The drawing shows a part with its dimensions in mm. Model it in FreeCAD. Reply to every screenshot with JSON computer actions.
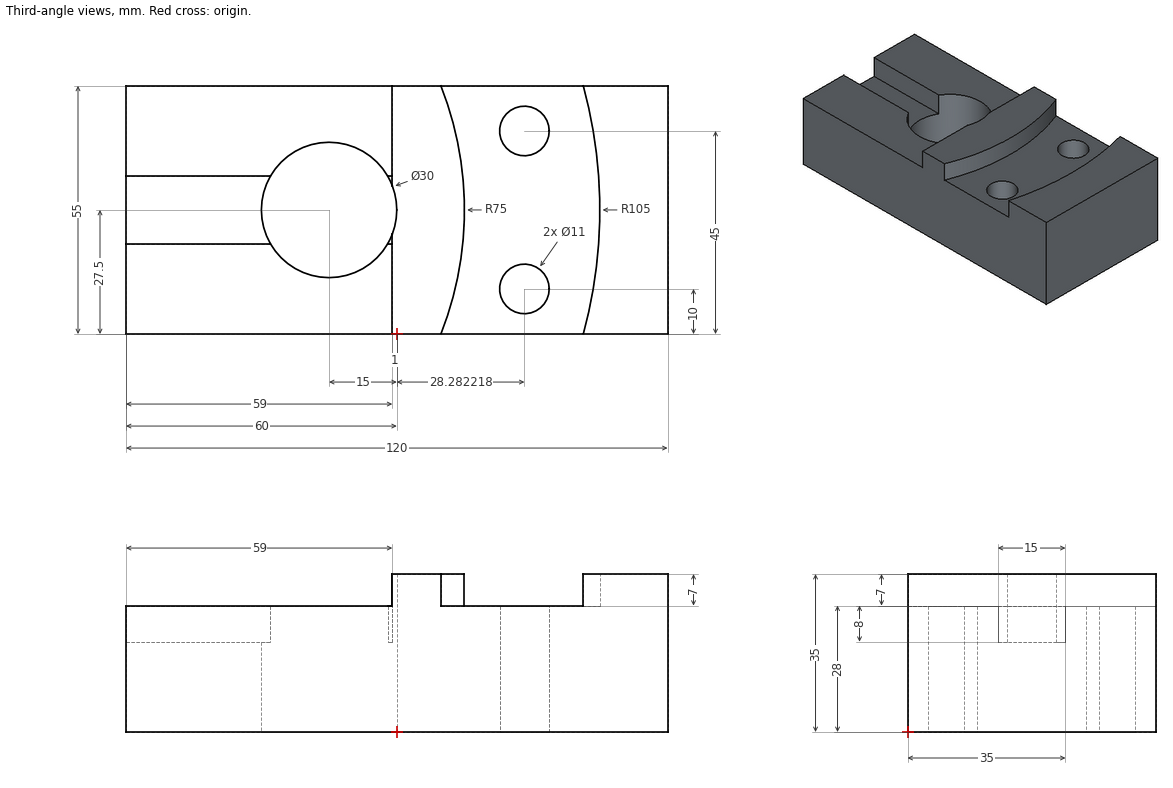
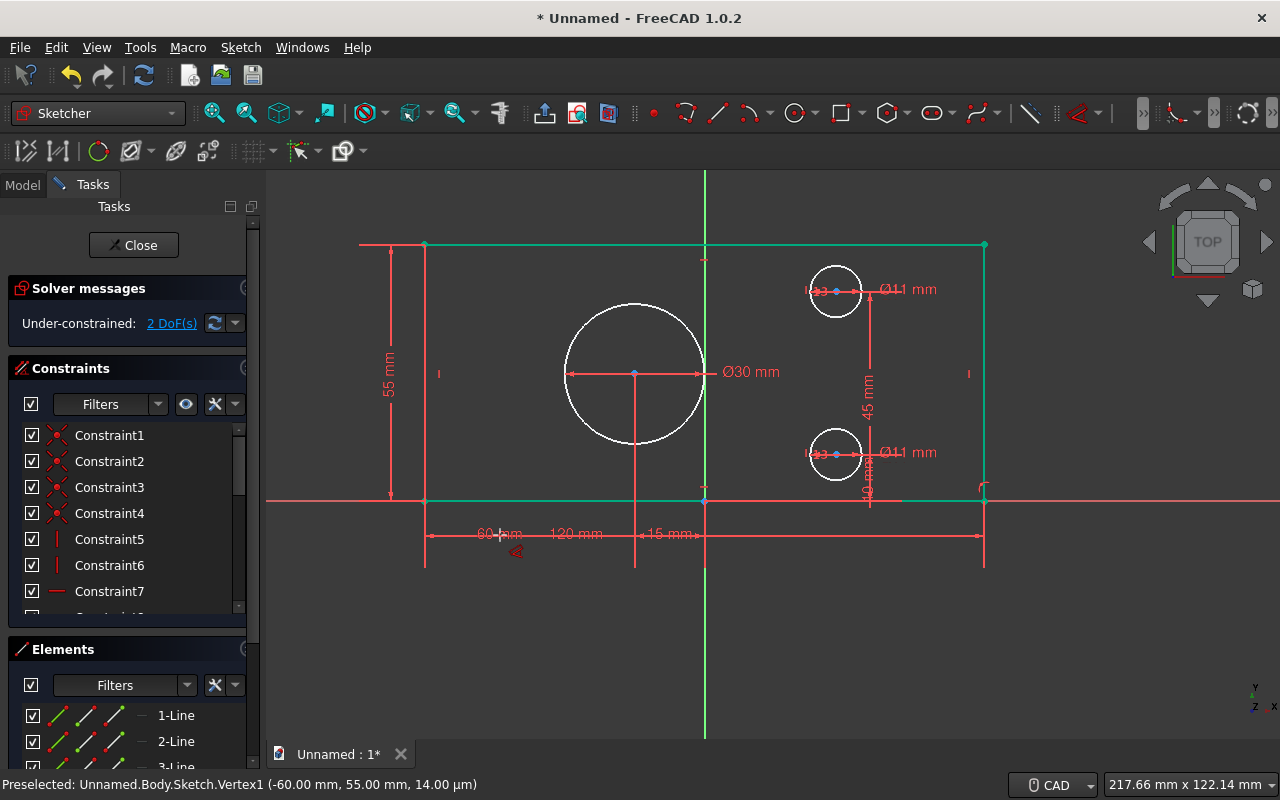
{"action": "left_click", "coordinate": [635, 374]}
{"action": "left_click", "coordinate": [601, 408]}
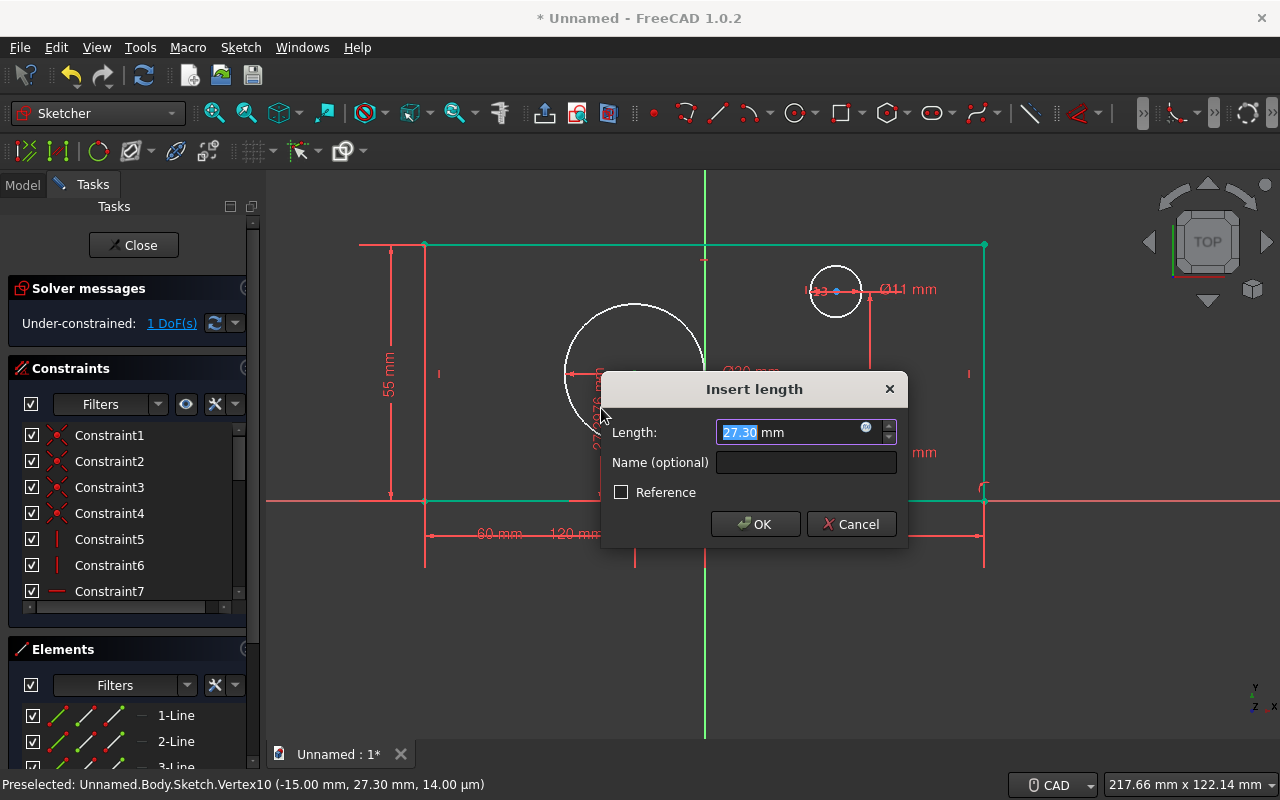
{"action": "type", "text": "27.5"}
{"action": "key", "text": "Return"}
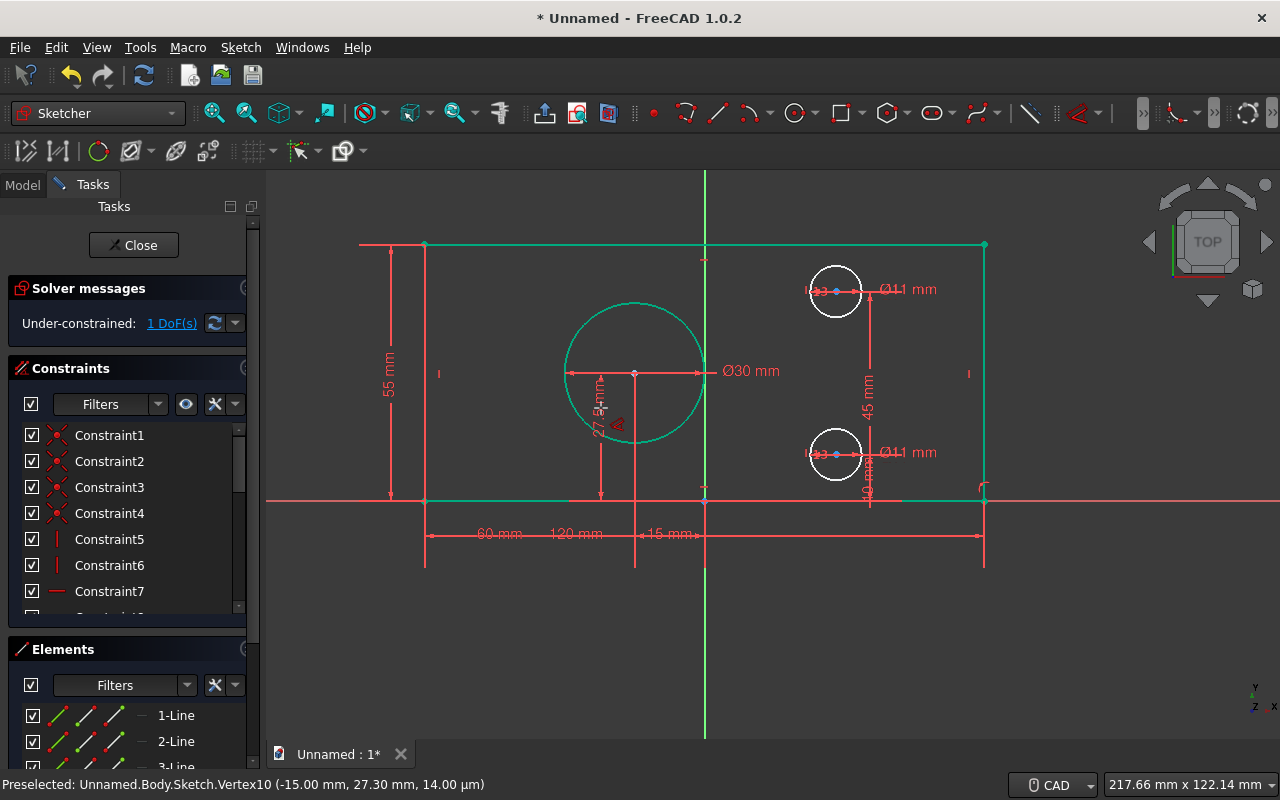
{"action": "left_click", "coordinate": [836, 455]}
{"action": "left_click", "coordinate": [770, 535]}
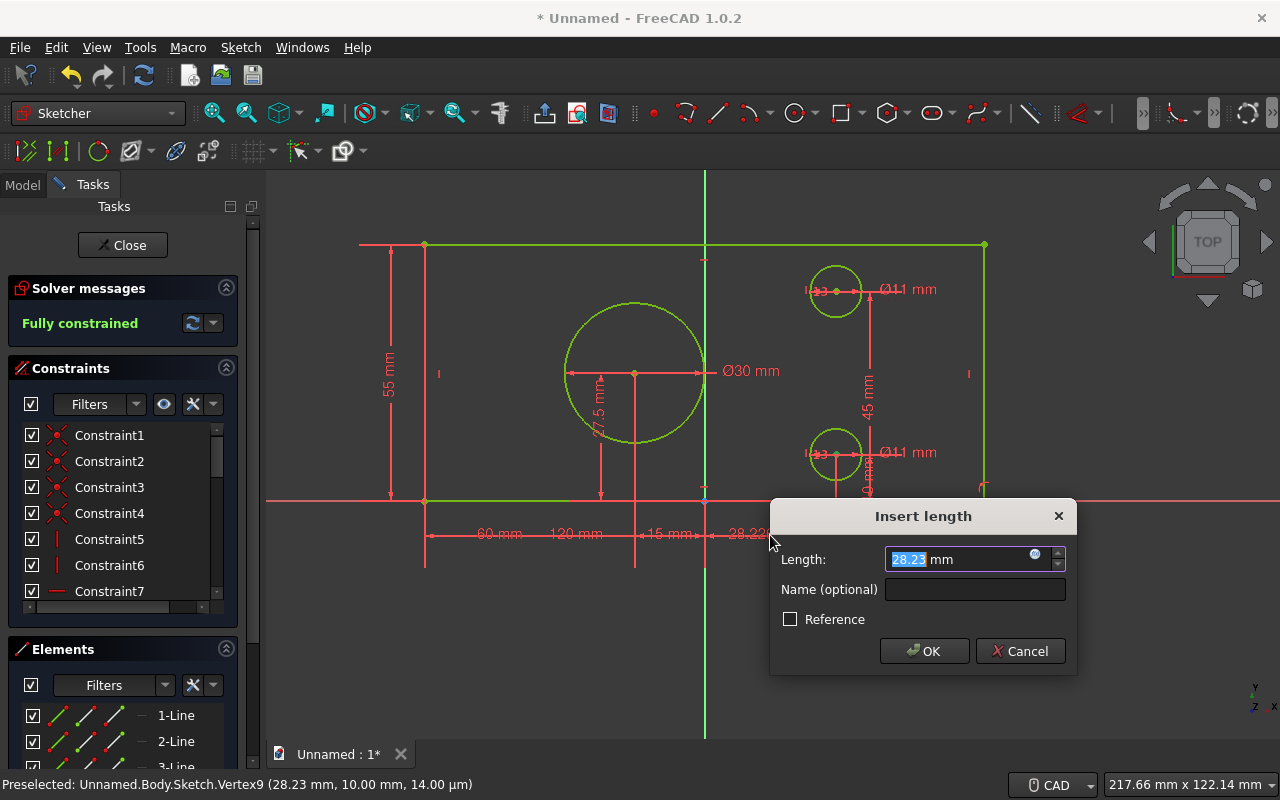
{"action": "type", "text": "28.282218"}
{"action": "key", "text": "Return"}
{"action": "key", "text": "Escape"}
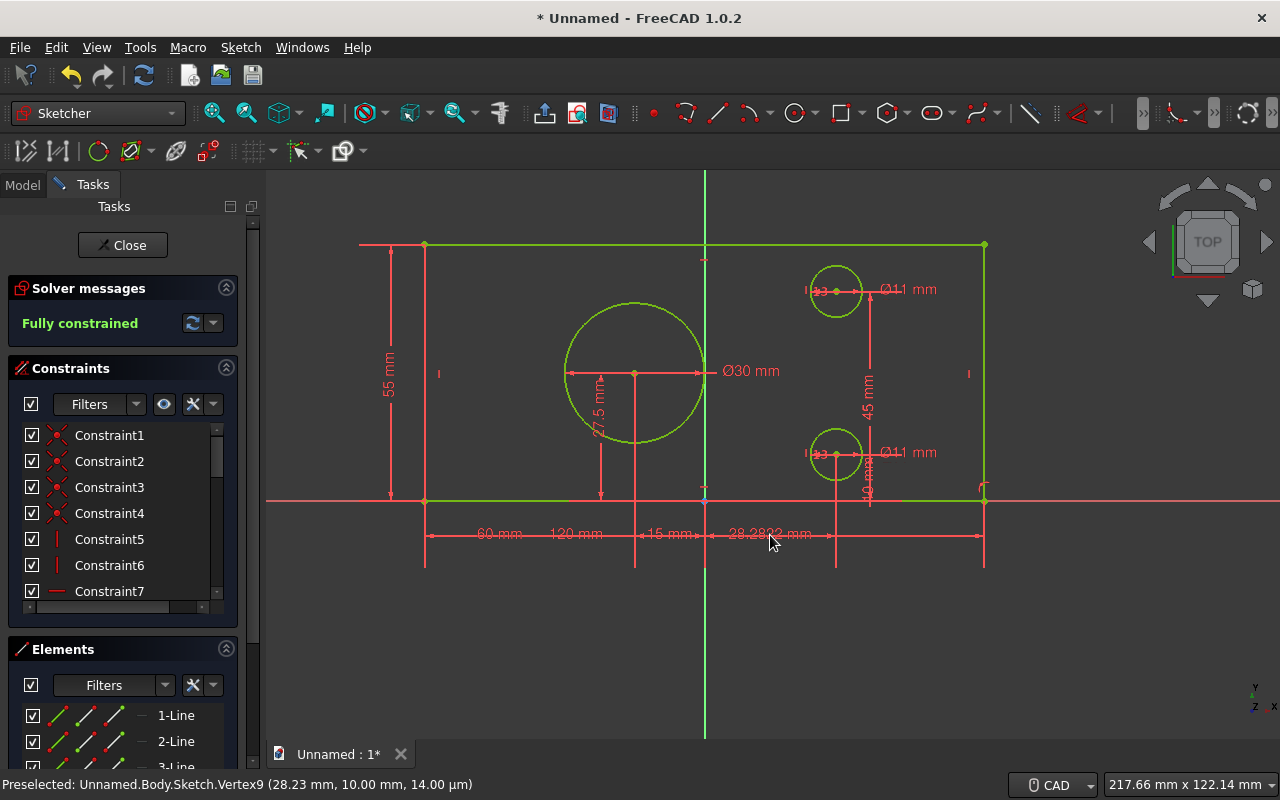
{"action": "left_click", "coordinate": [123, 245]}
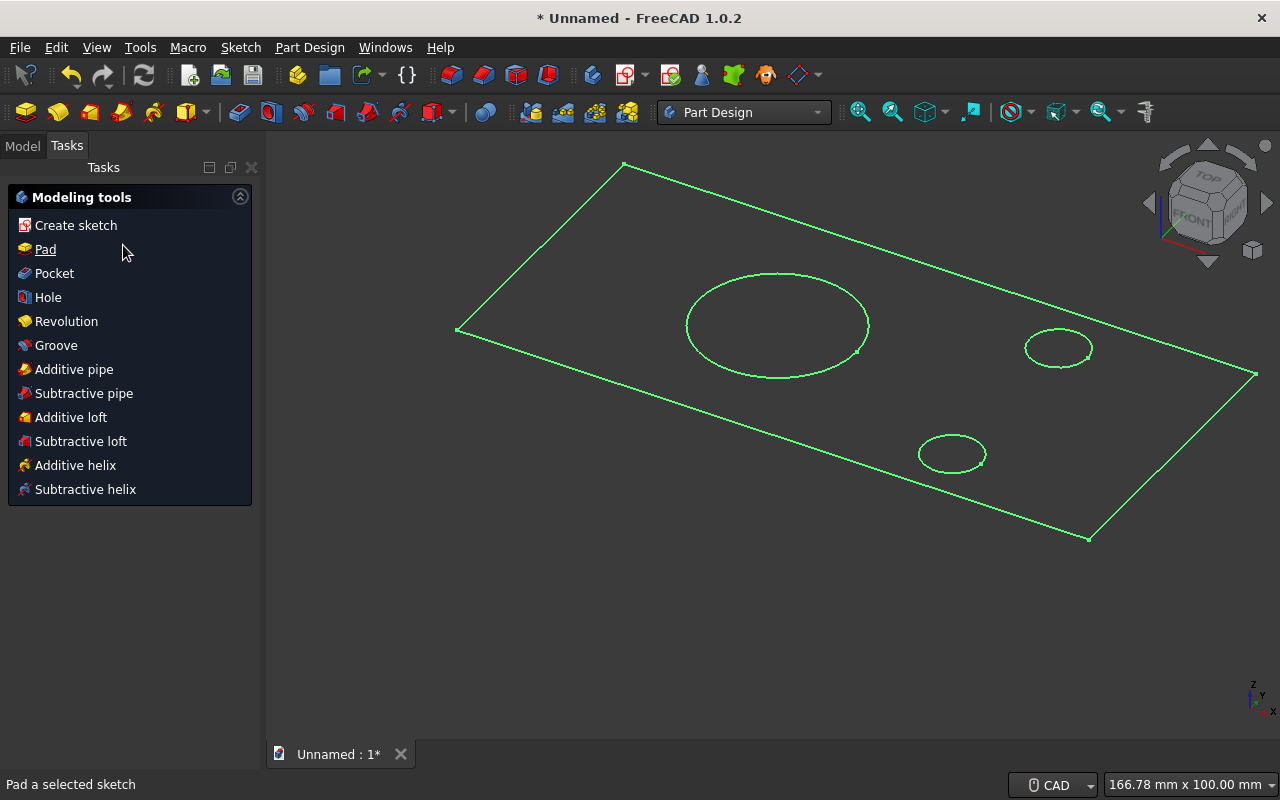
{"action": "left_click", "coordinate": [26, 112]}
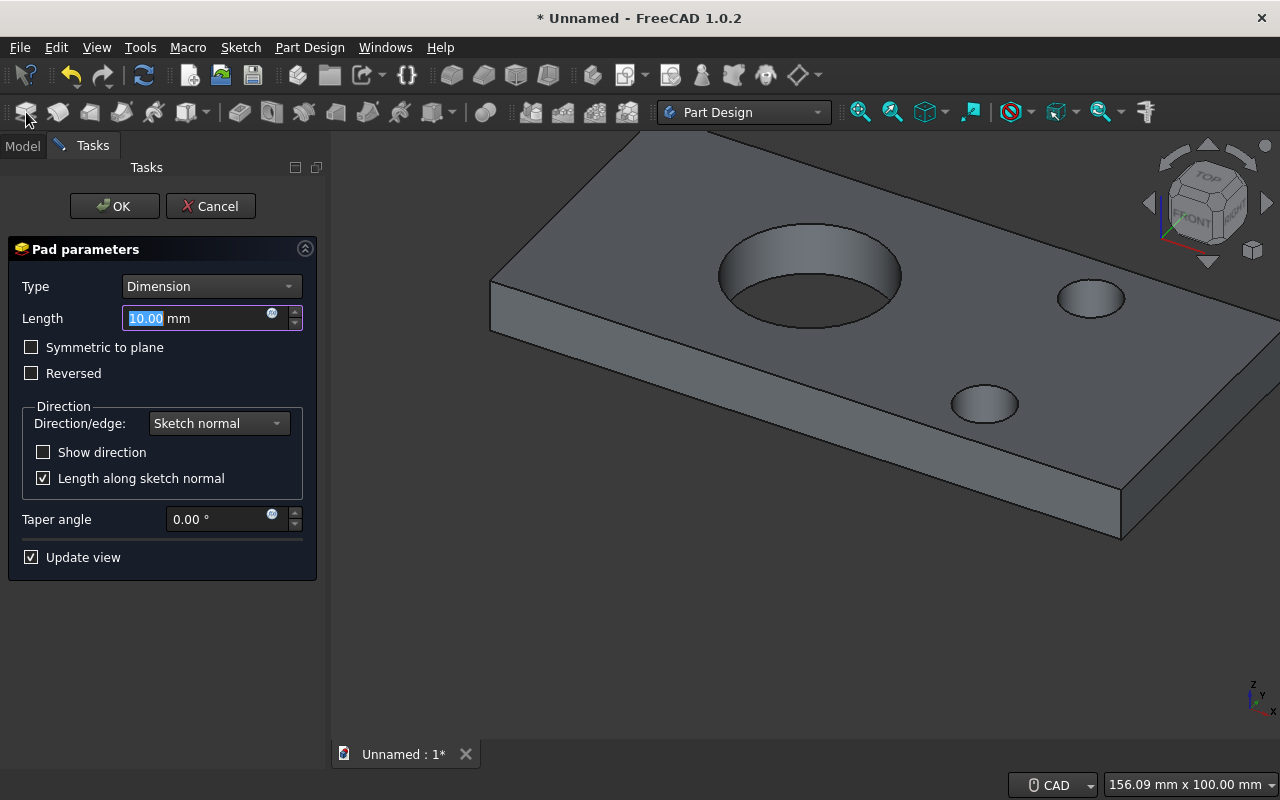
{"action": "type", "text": "35"}
{"action": "key", "text": "Tab"}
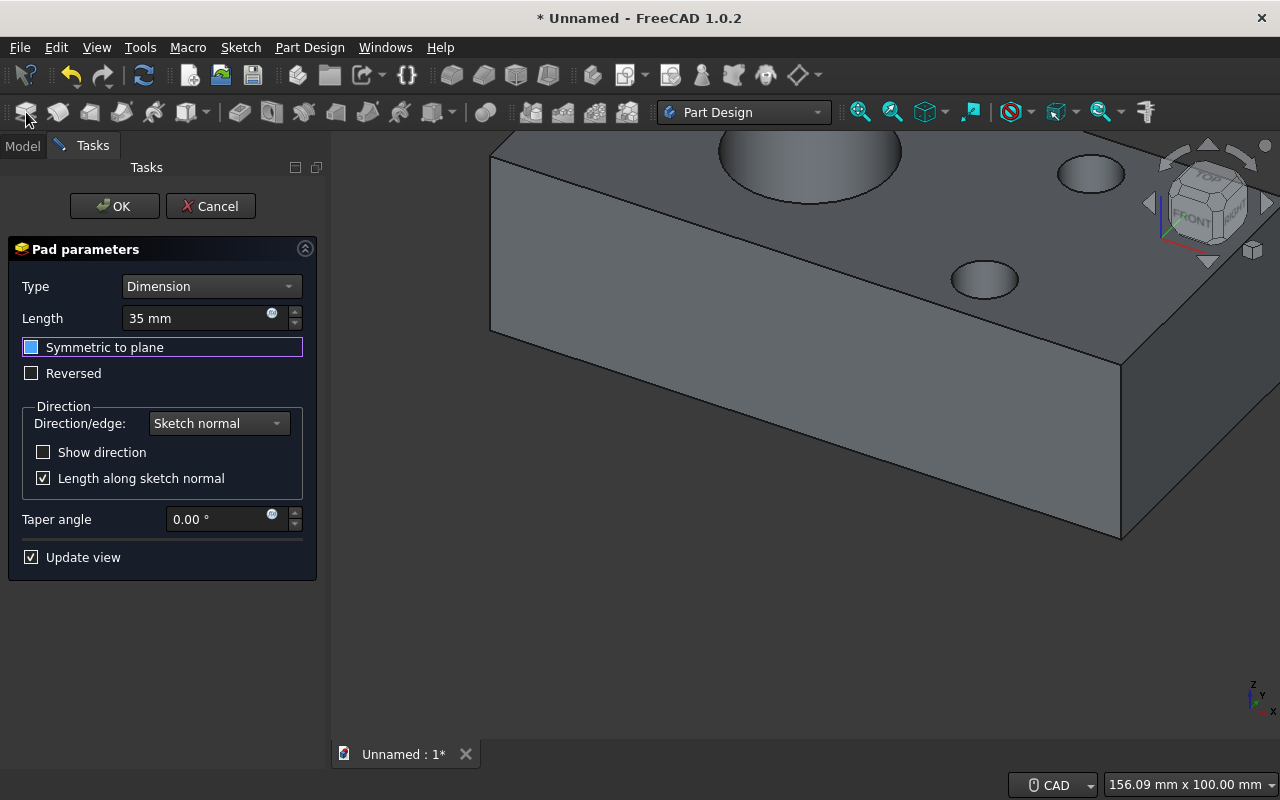
{"action": "left_click", "coordinate": [115, 206]}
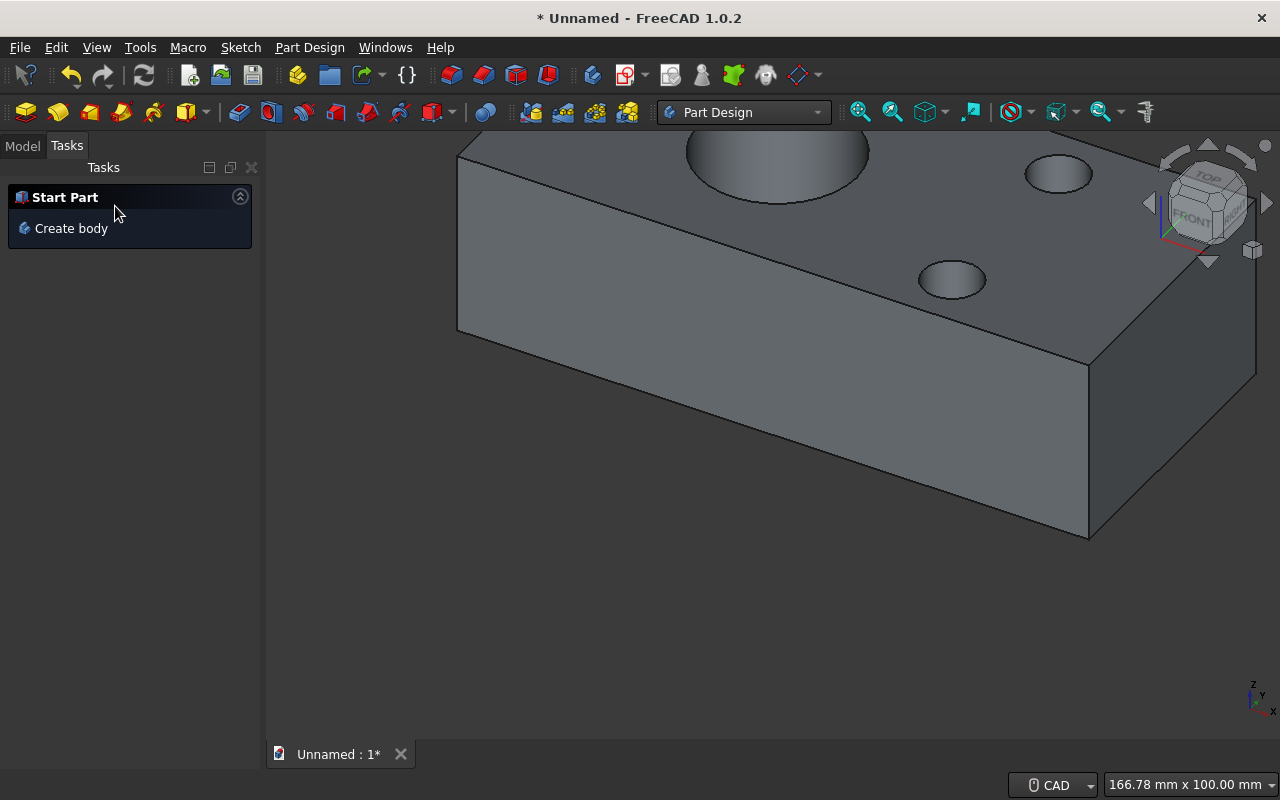
{"action": "left_click", "coordinate": [862, 112]}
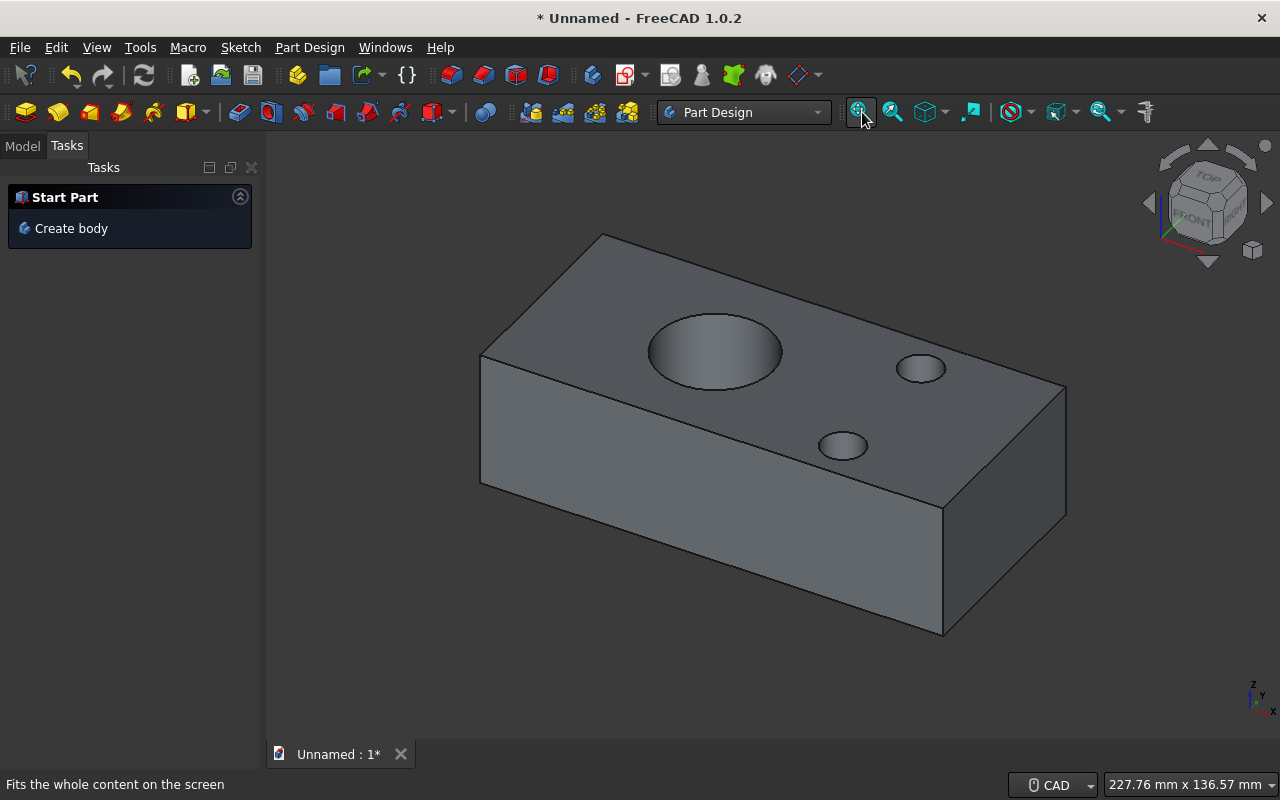
{"action": "left_click", "coordinate": [839, 392]}